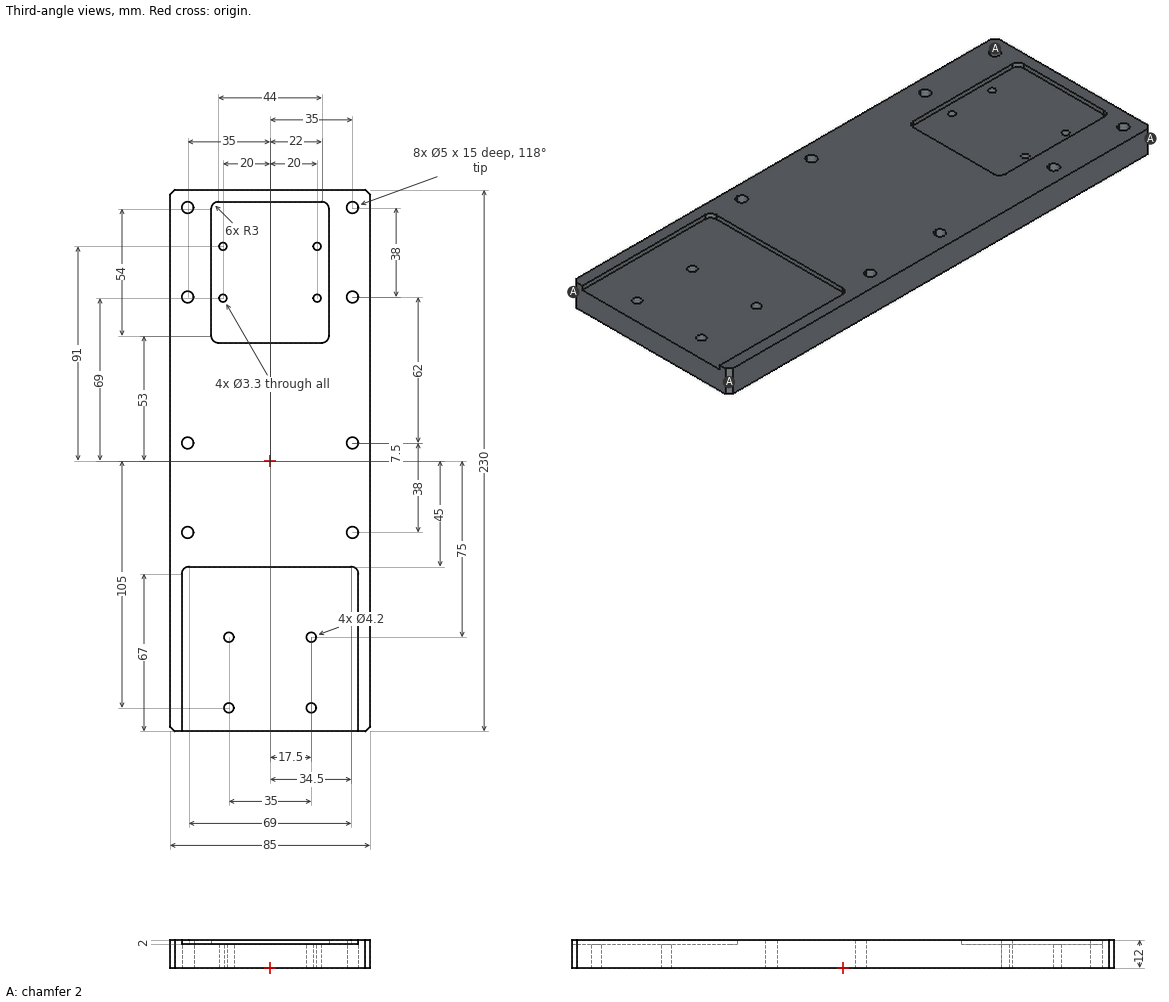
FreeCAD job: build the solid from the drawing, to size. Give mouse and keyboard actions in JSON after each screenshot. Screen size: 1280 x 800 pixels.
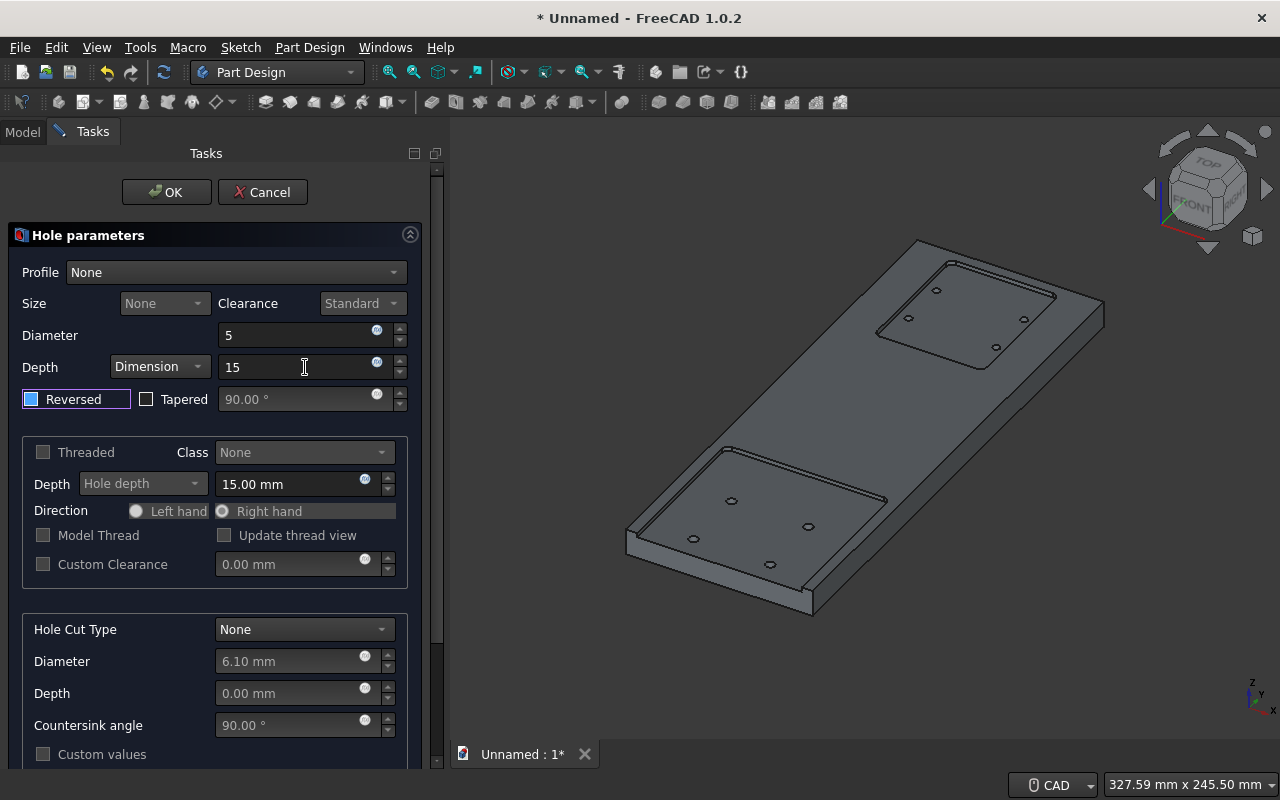
{"action": "left_click", "coordinate": [30, 399]}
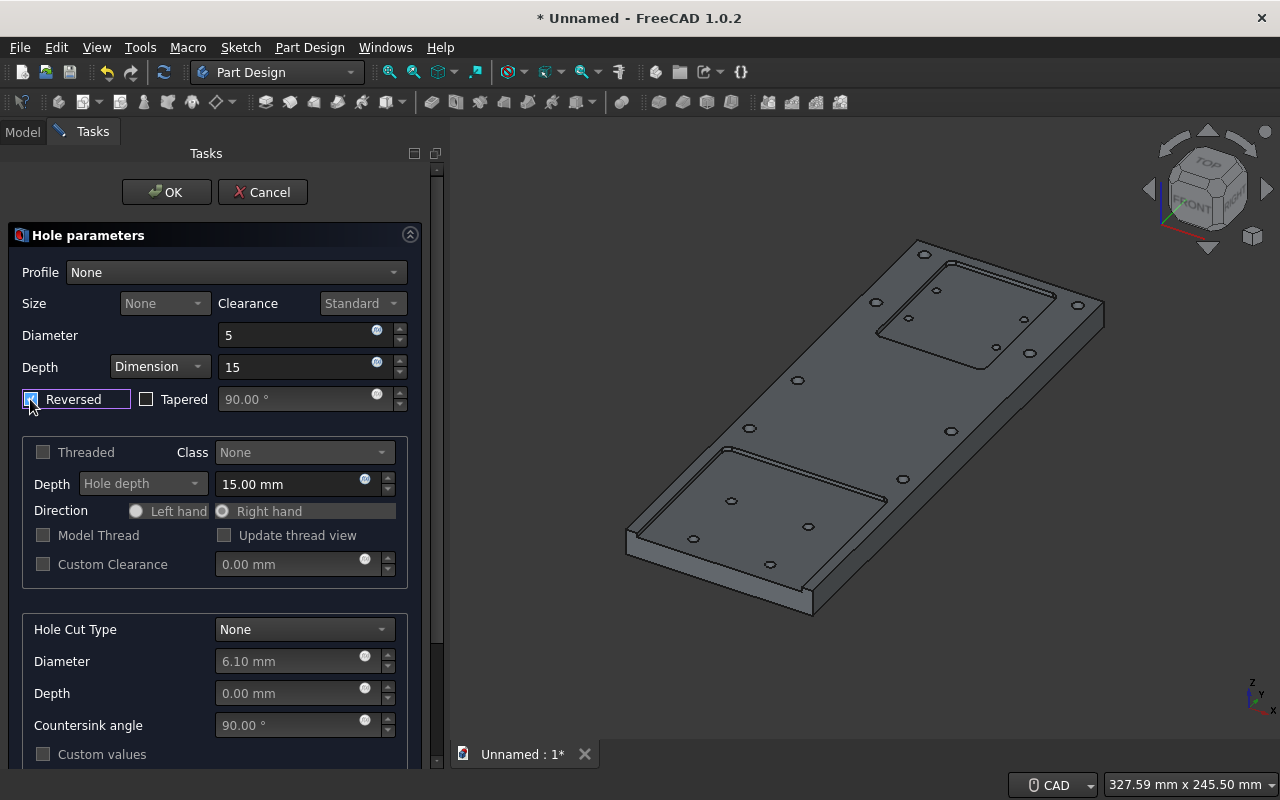
{"action": "left_click", "coordinate": [167, 192]}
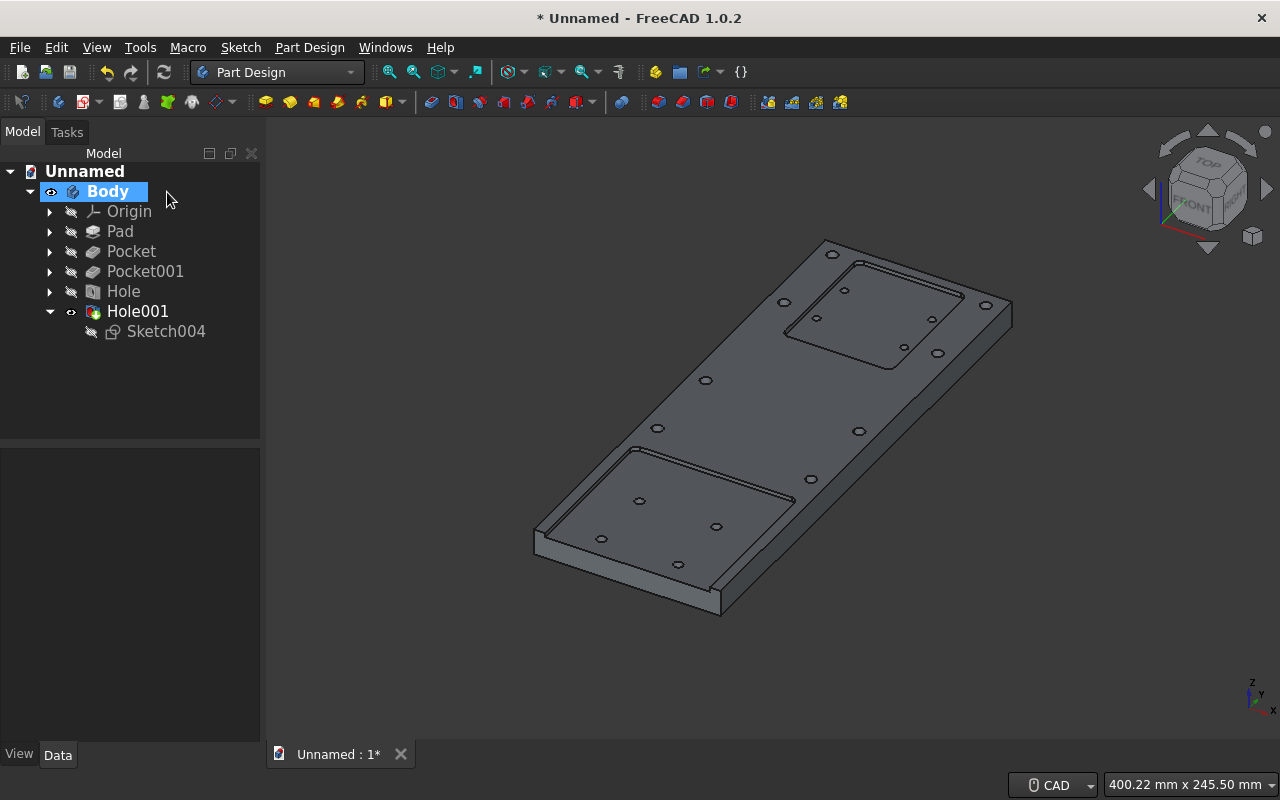
{"action": "left_click", "coordinate": [721, 603]}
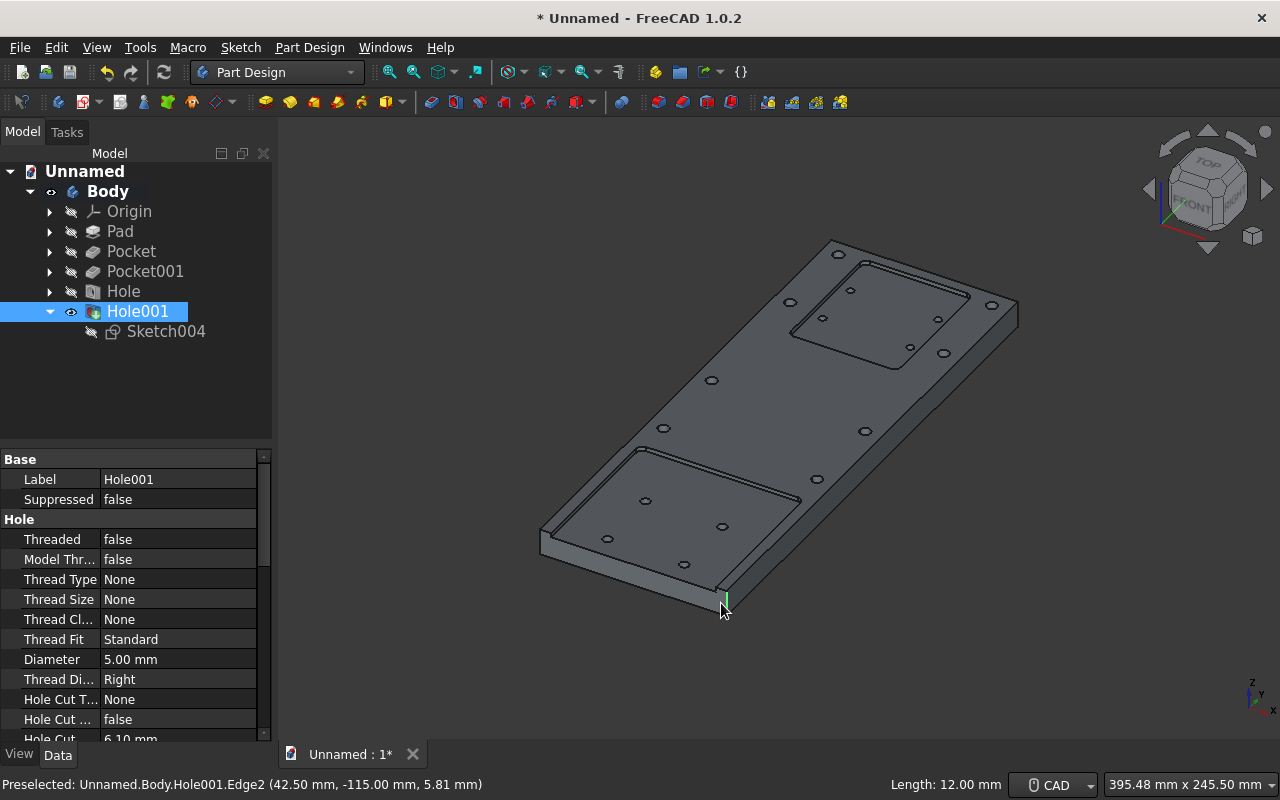
{"action": "key", "text": "0"}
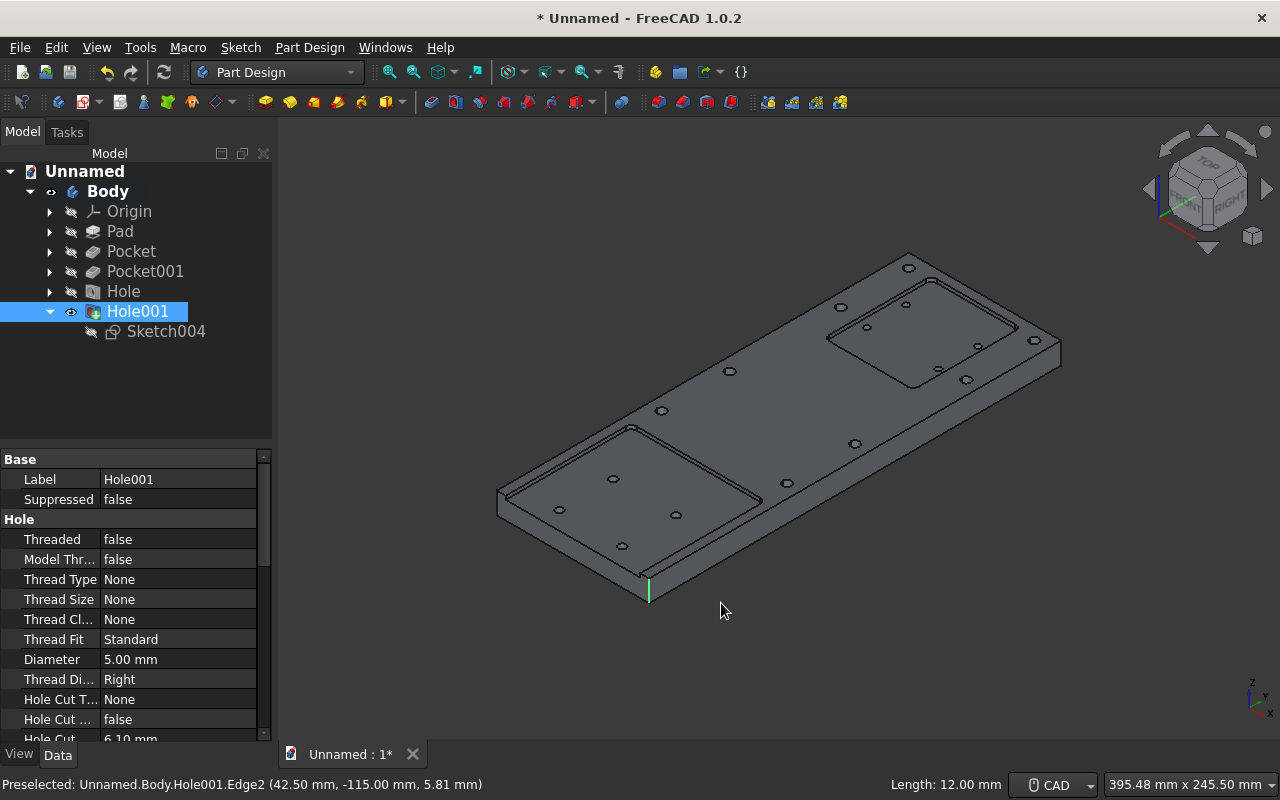
{"action": "key", "text": "2"}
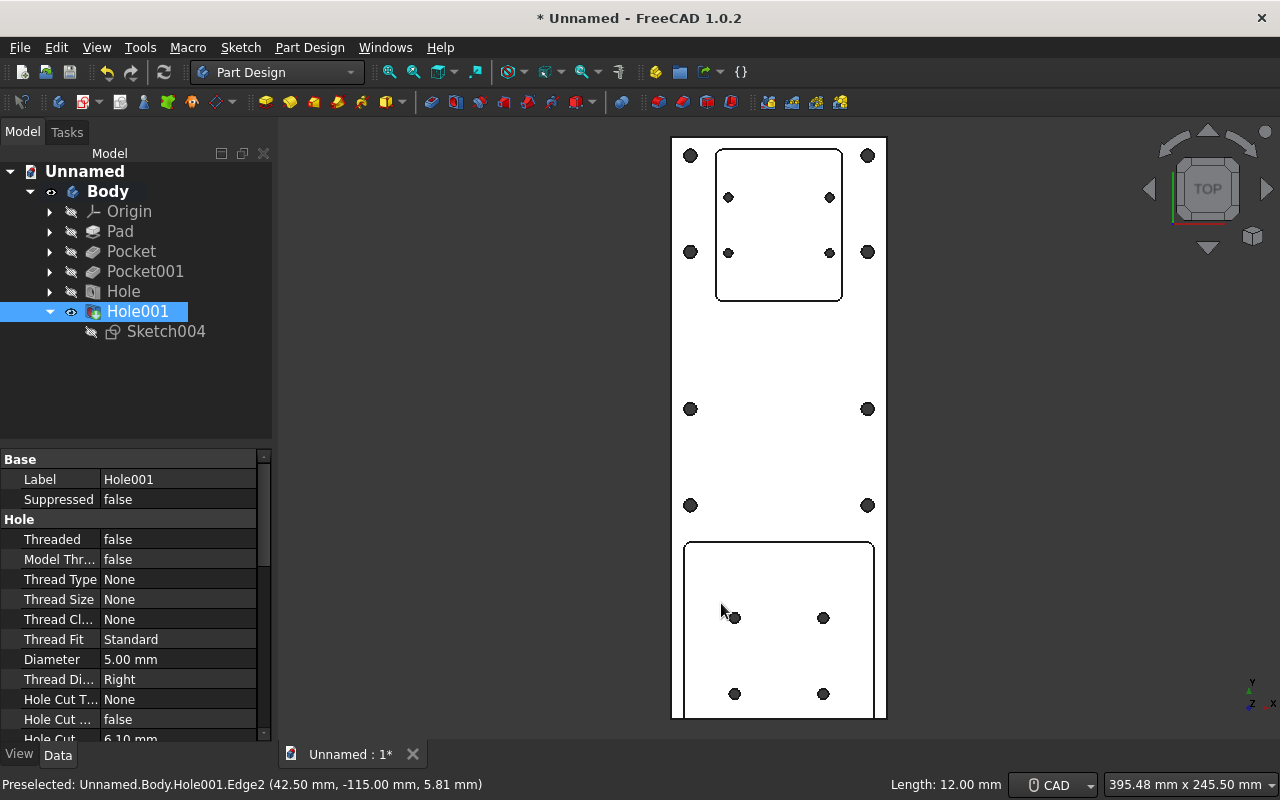
{"action": "key", "text": "1"}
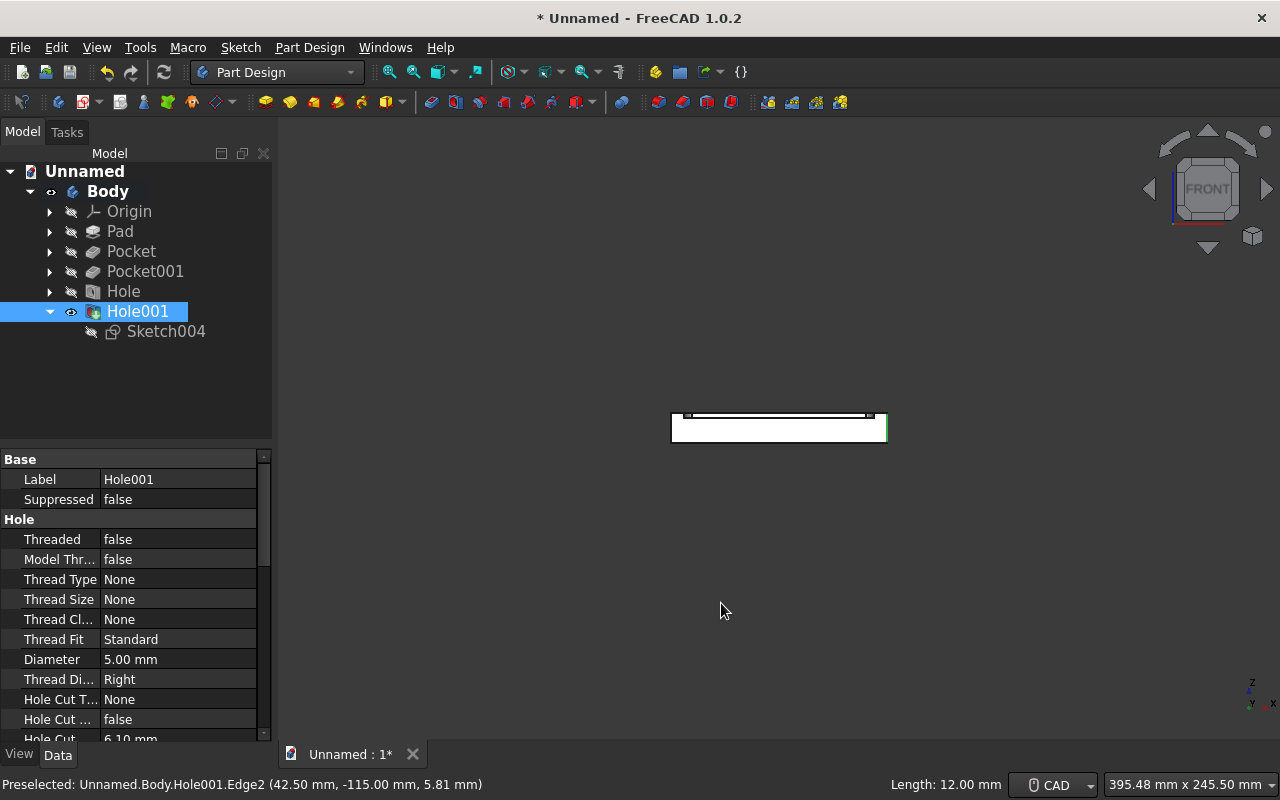
{"action": "left_click", "coordinate": [390, 72]}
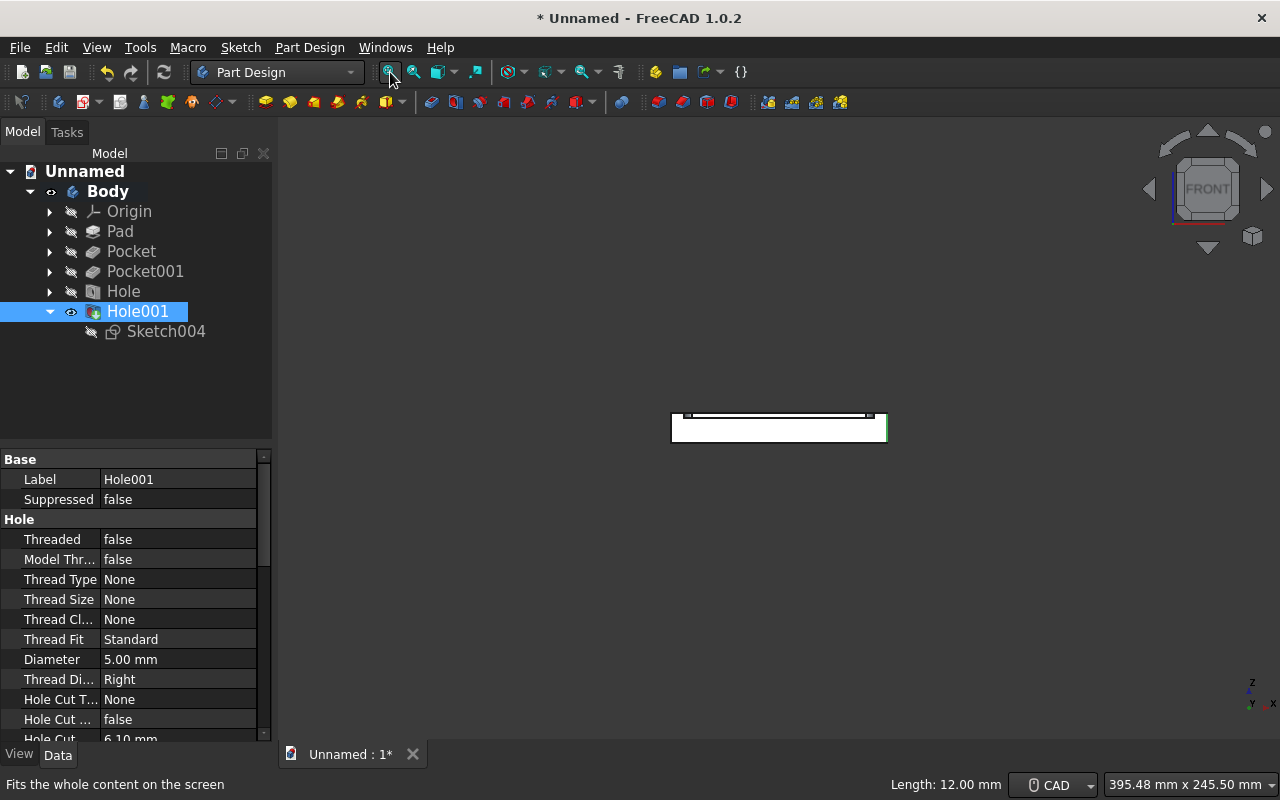
{"action": "left_click", "coordinate": [671, 427], "text": "ctrl"}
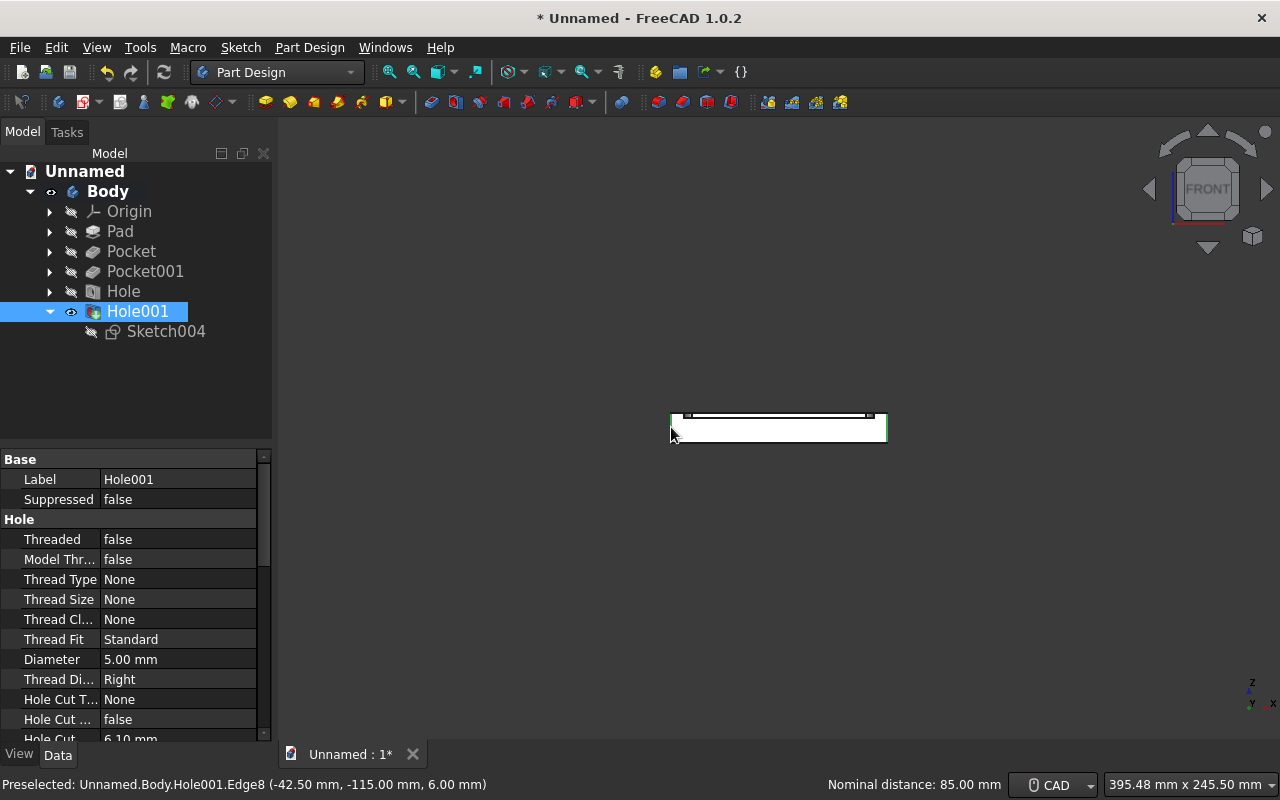
{"action": "key", "text": "3"}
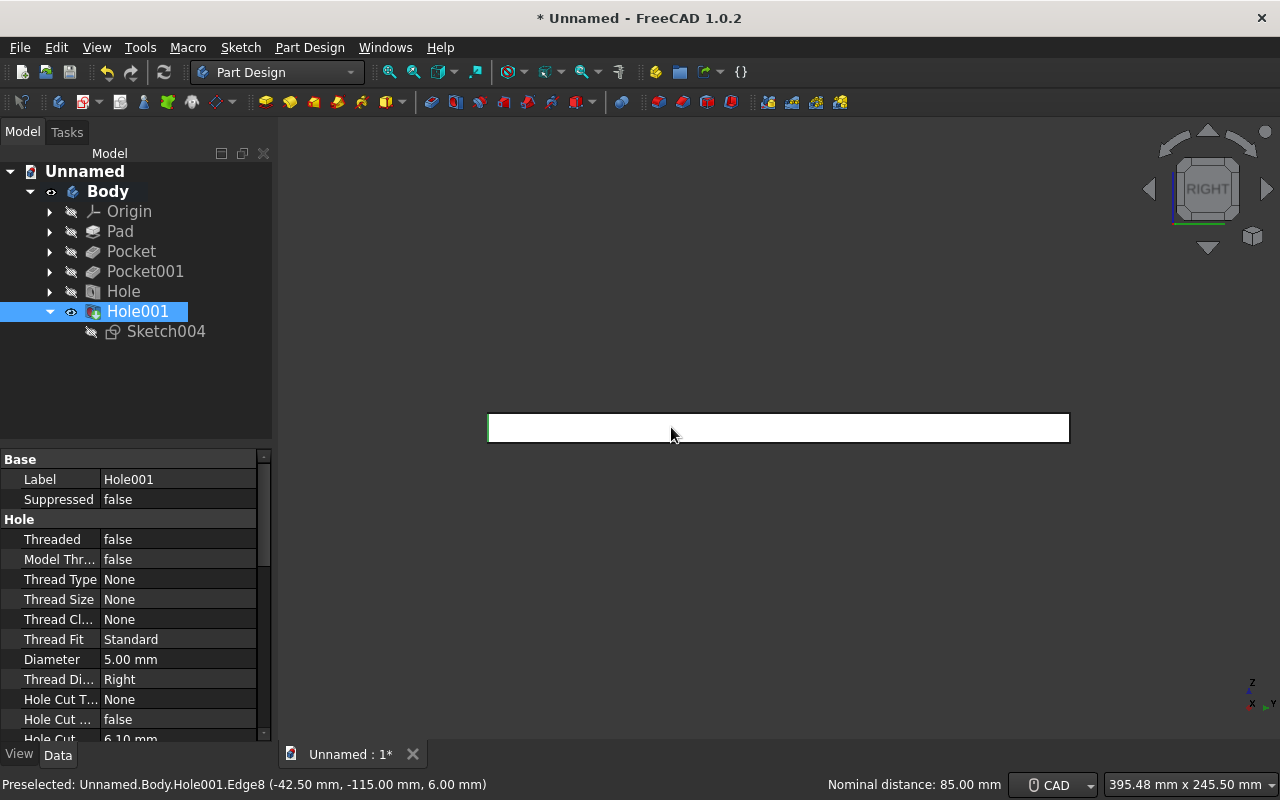
{"action": "left_click", "coordinate": [1070, 427], "text": "ctrl"}